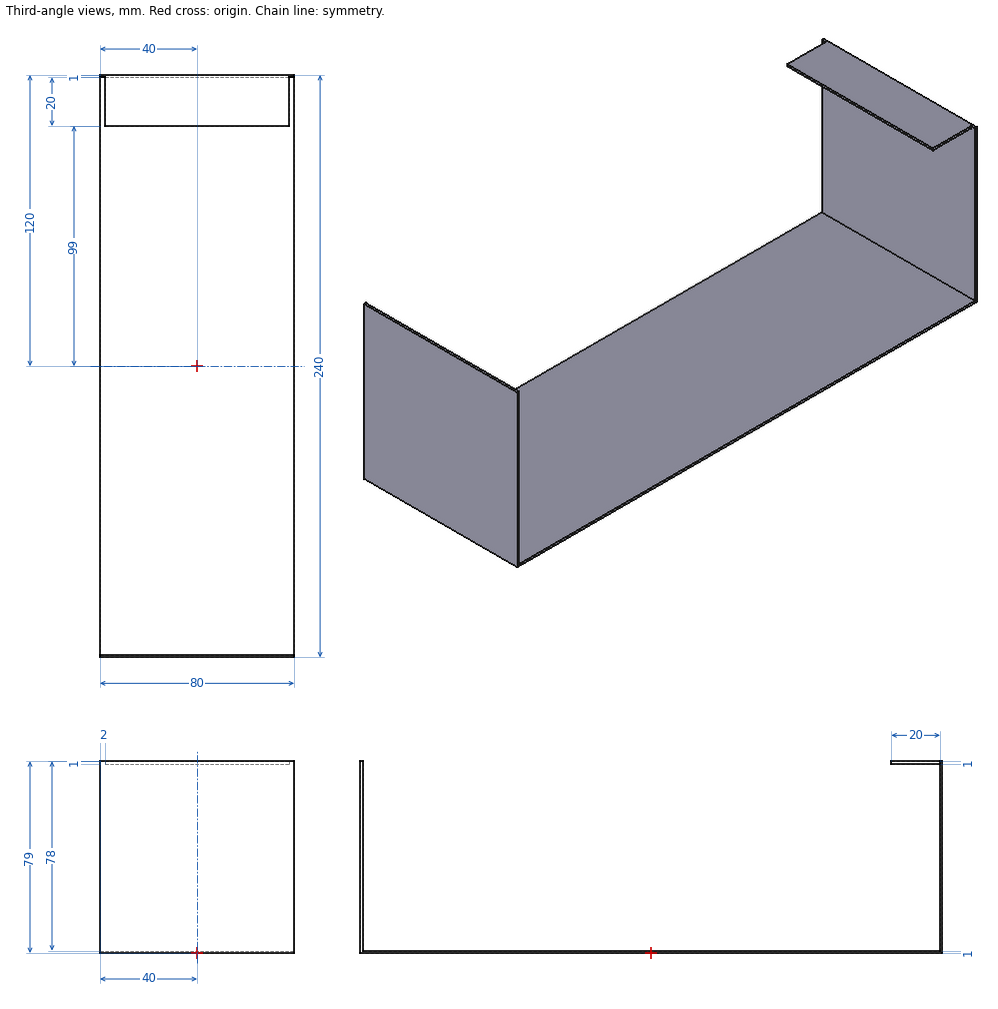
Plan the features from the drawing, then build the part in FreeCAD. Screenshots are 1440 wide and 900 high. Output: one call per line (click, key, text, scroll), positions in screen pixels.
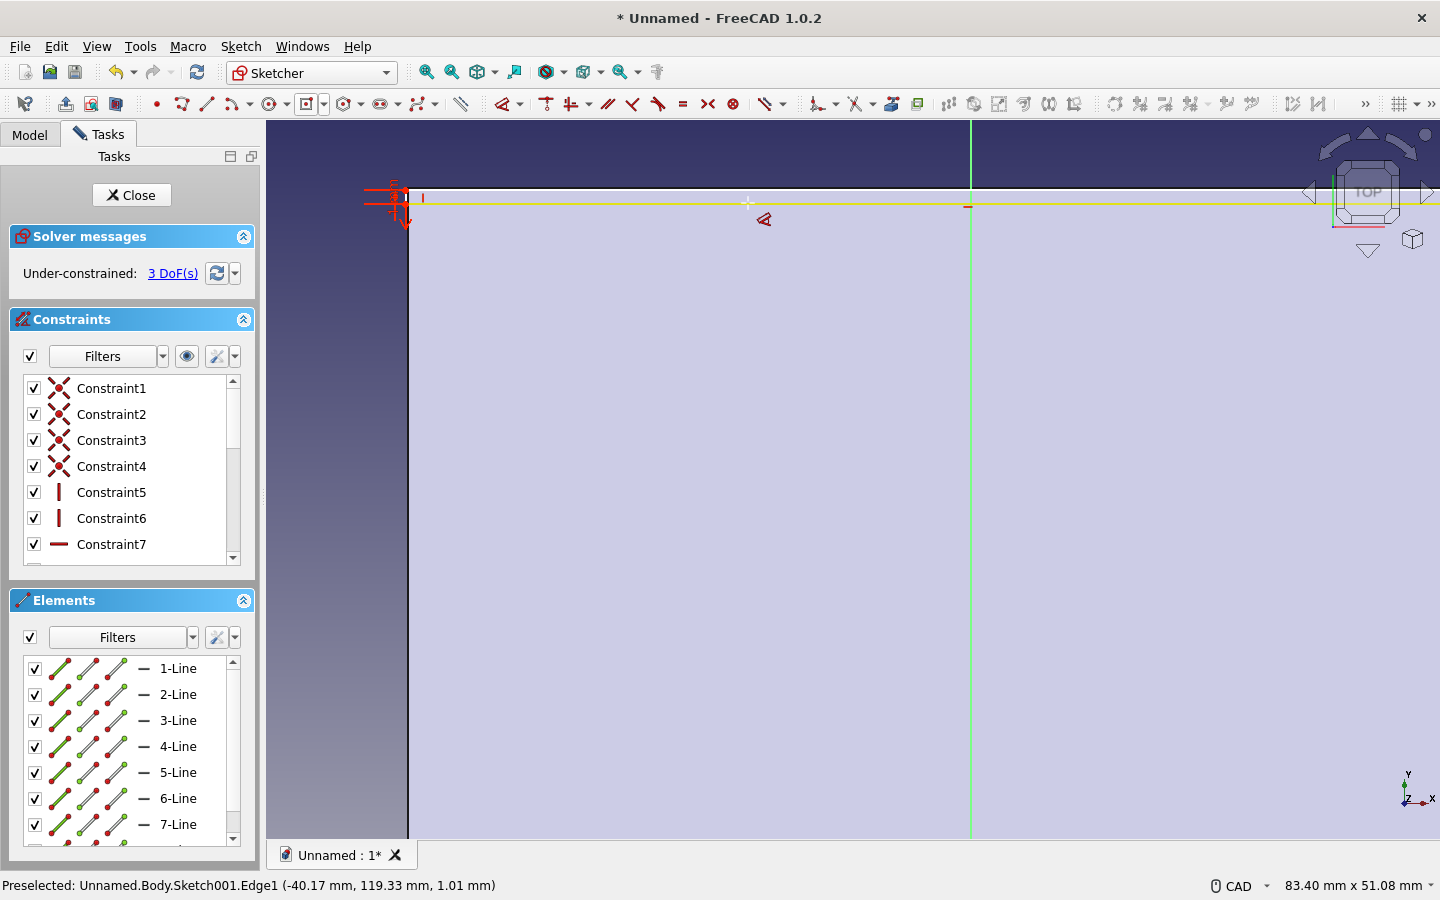
click(745, 204)
click(840, 170)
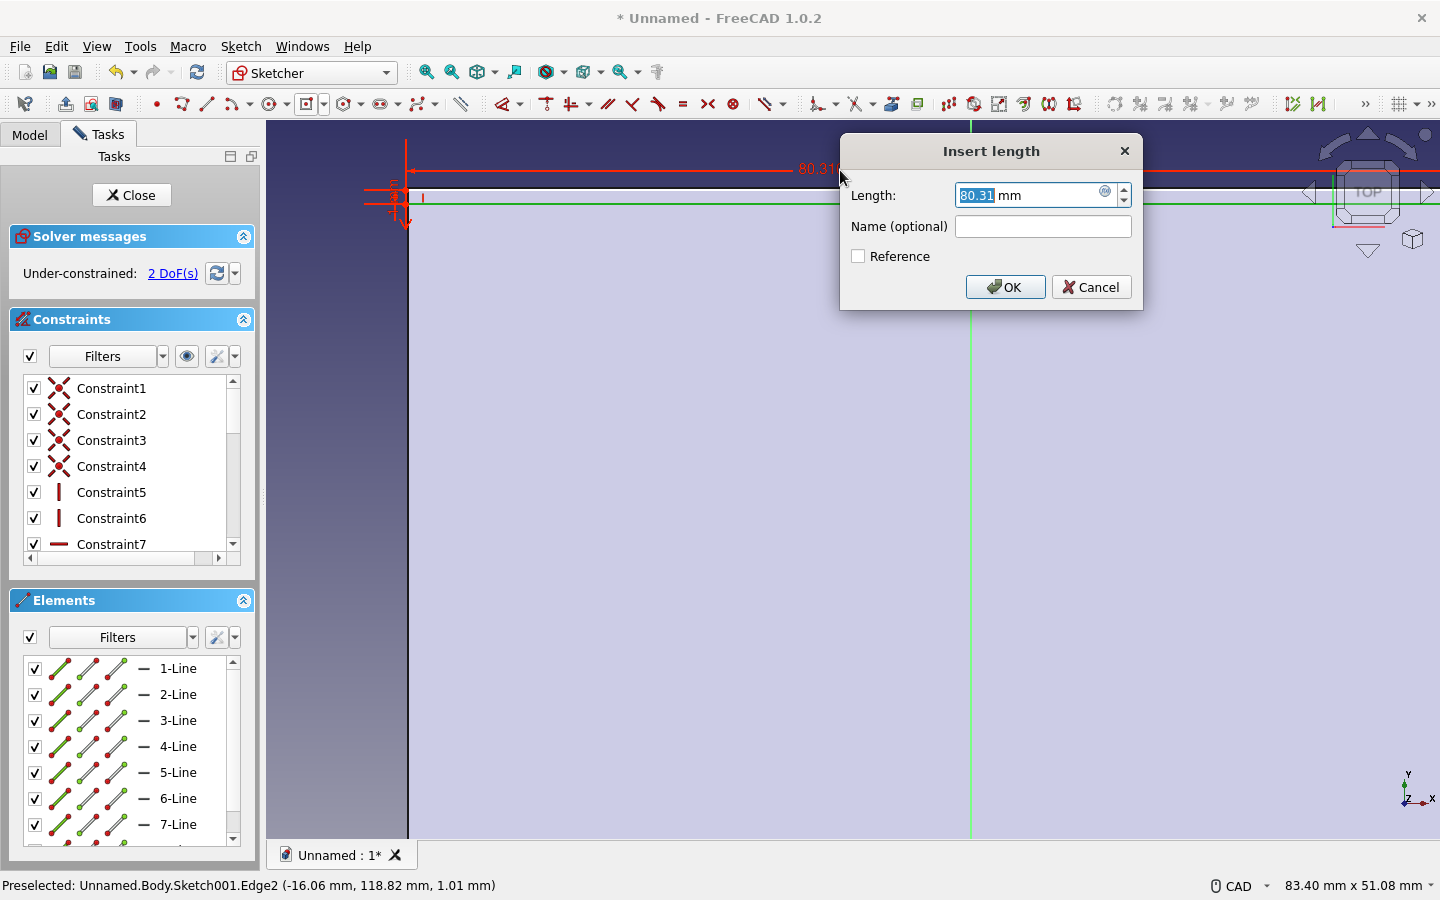
text(80)
key(Return)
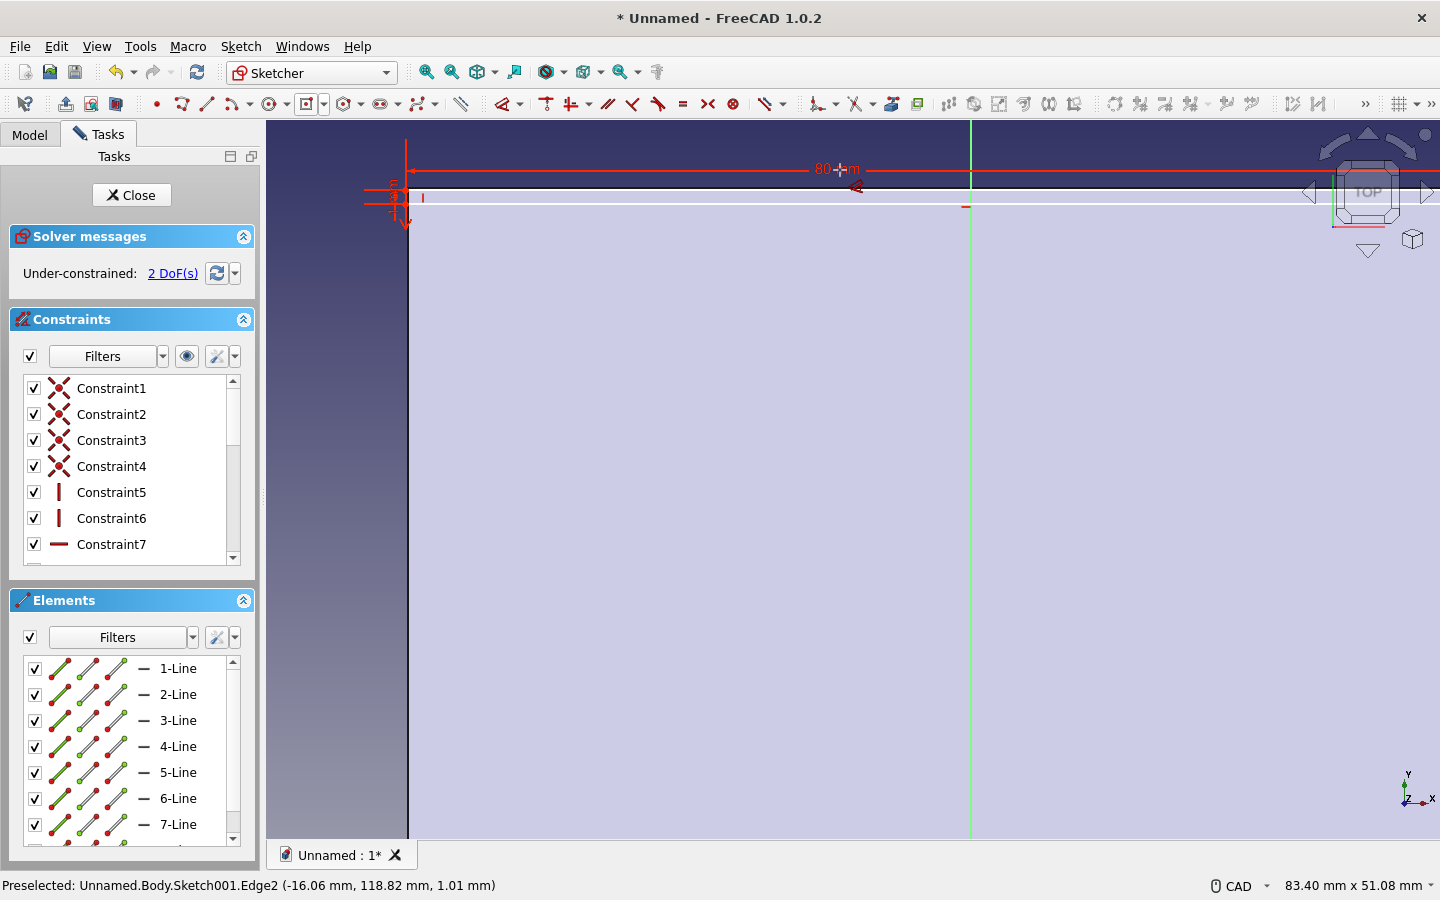
click(406, 190)
click(688, 156)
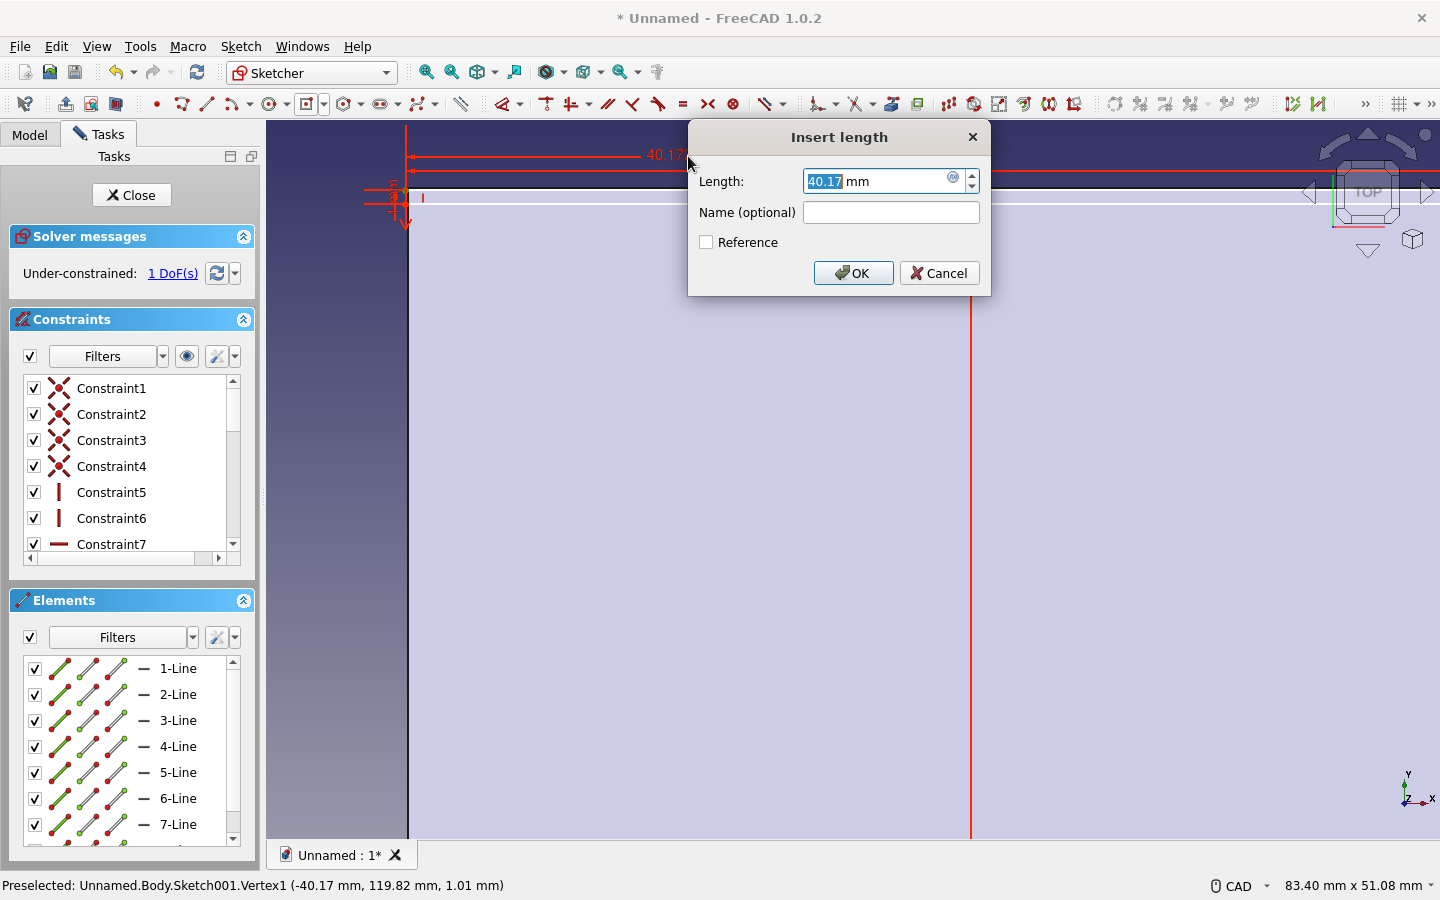
text(40)
key(Return)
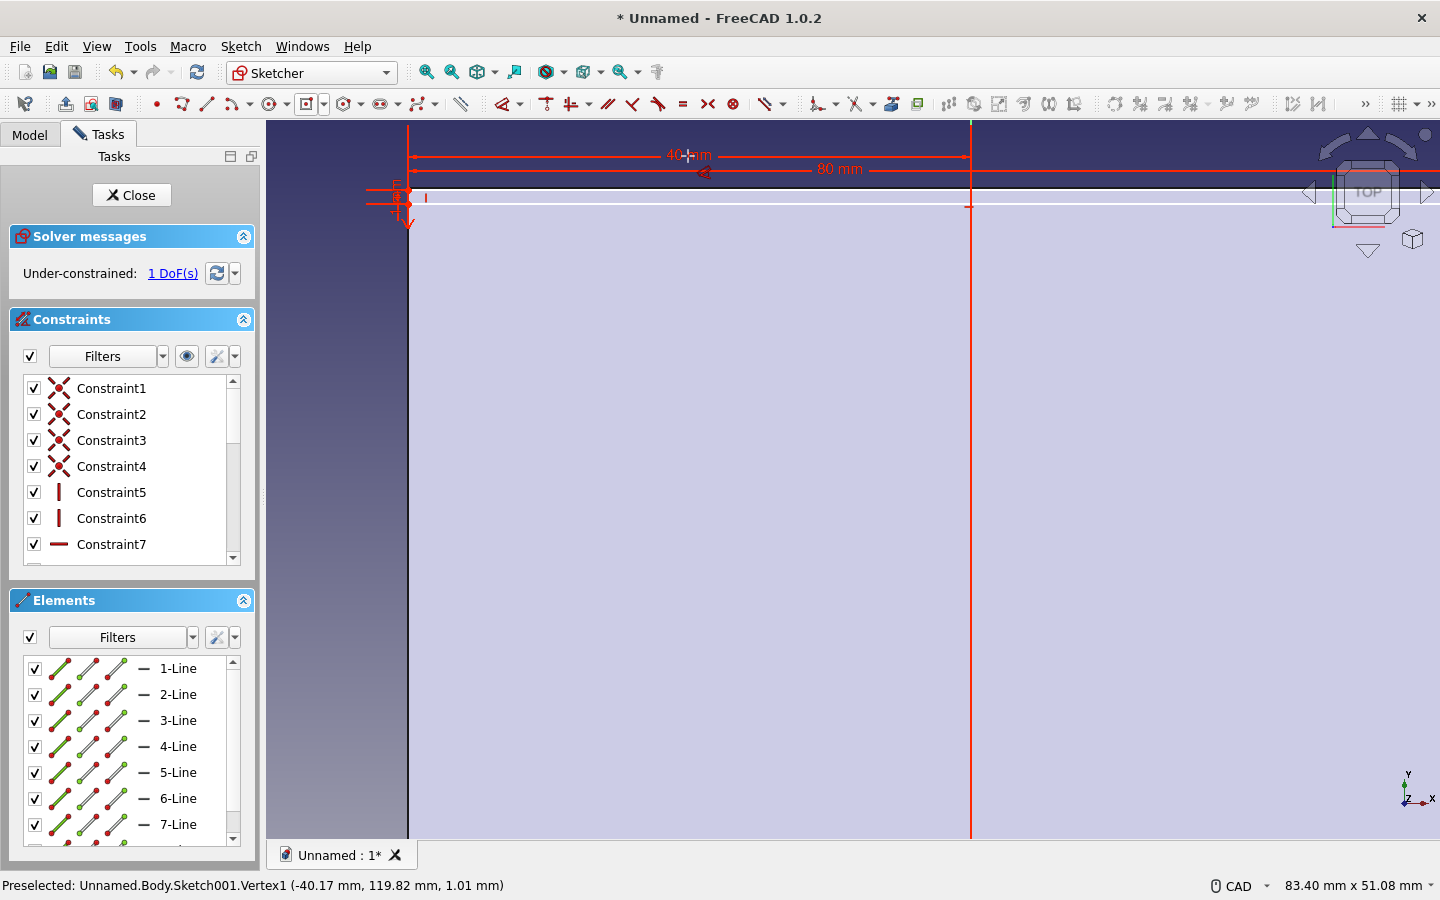
click(408, 190)
click(374, 501)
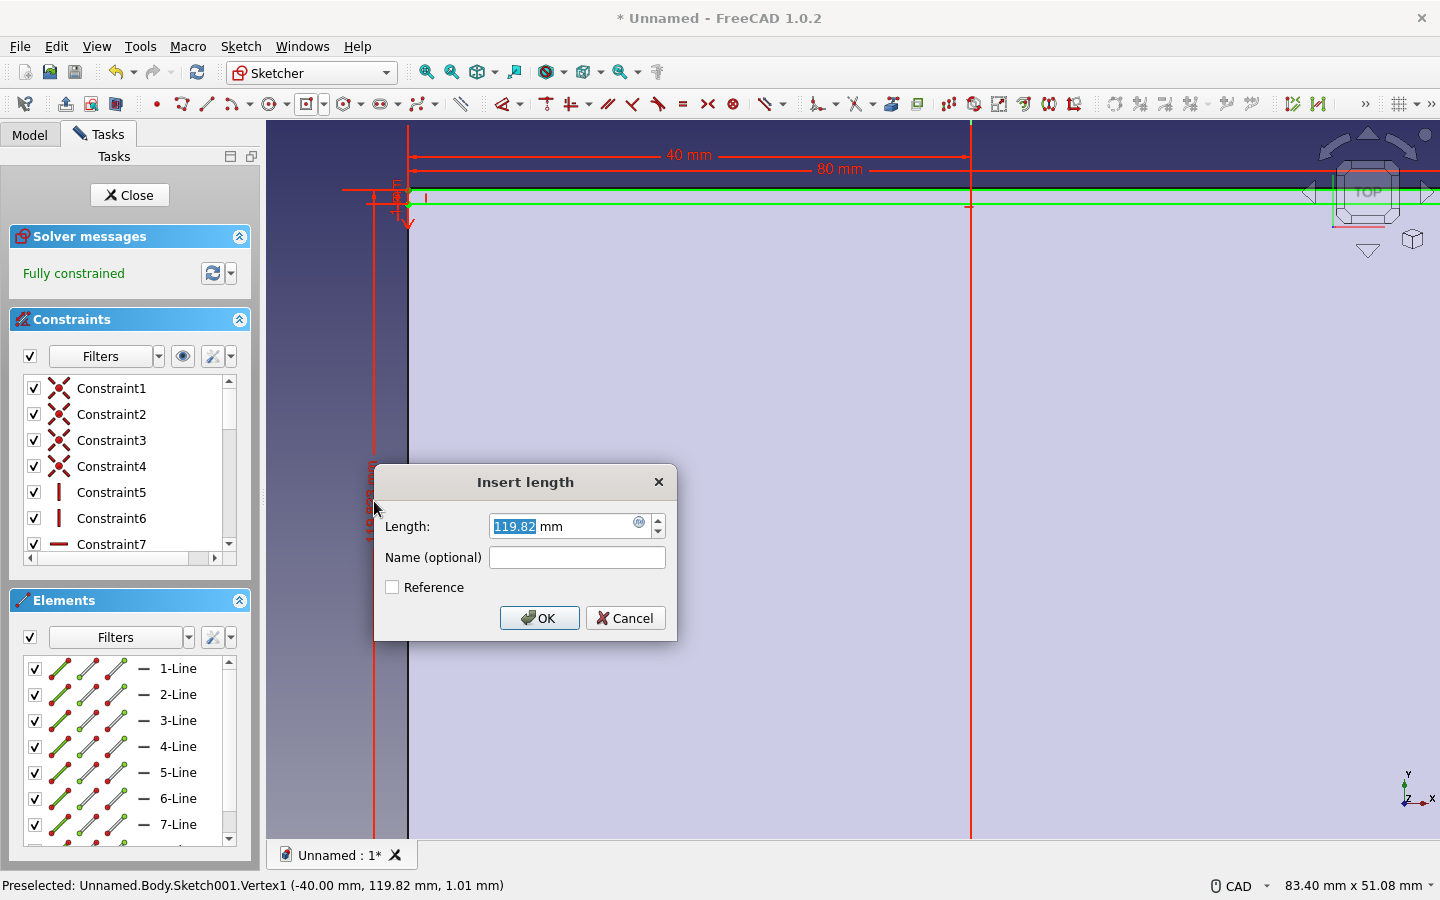
text(120)
key(Return)
key(Escape)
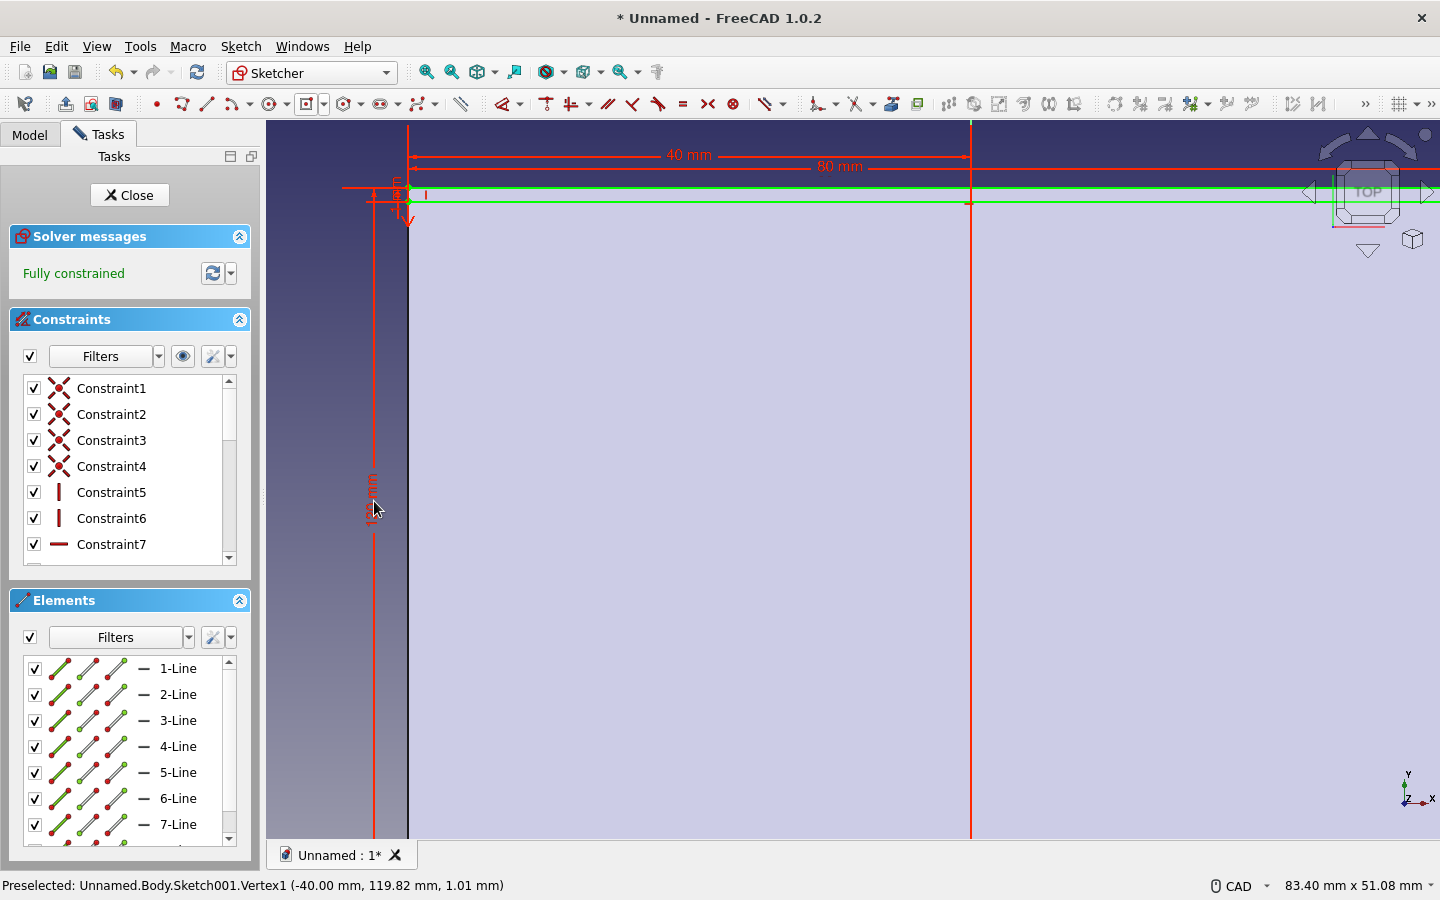
click(130, 195)